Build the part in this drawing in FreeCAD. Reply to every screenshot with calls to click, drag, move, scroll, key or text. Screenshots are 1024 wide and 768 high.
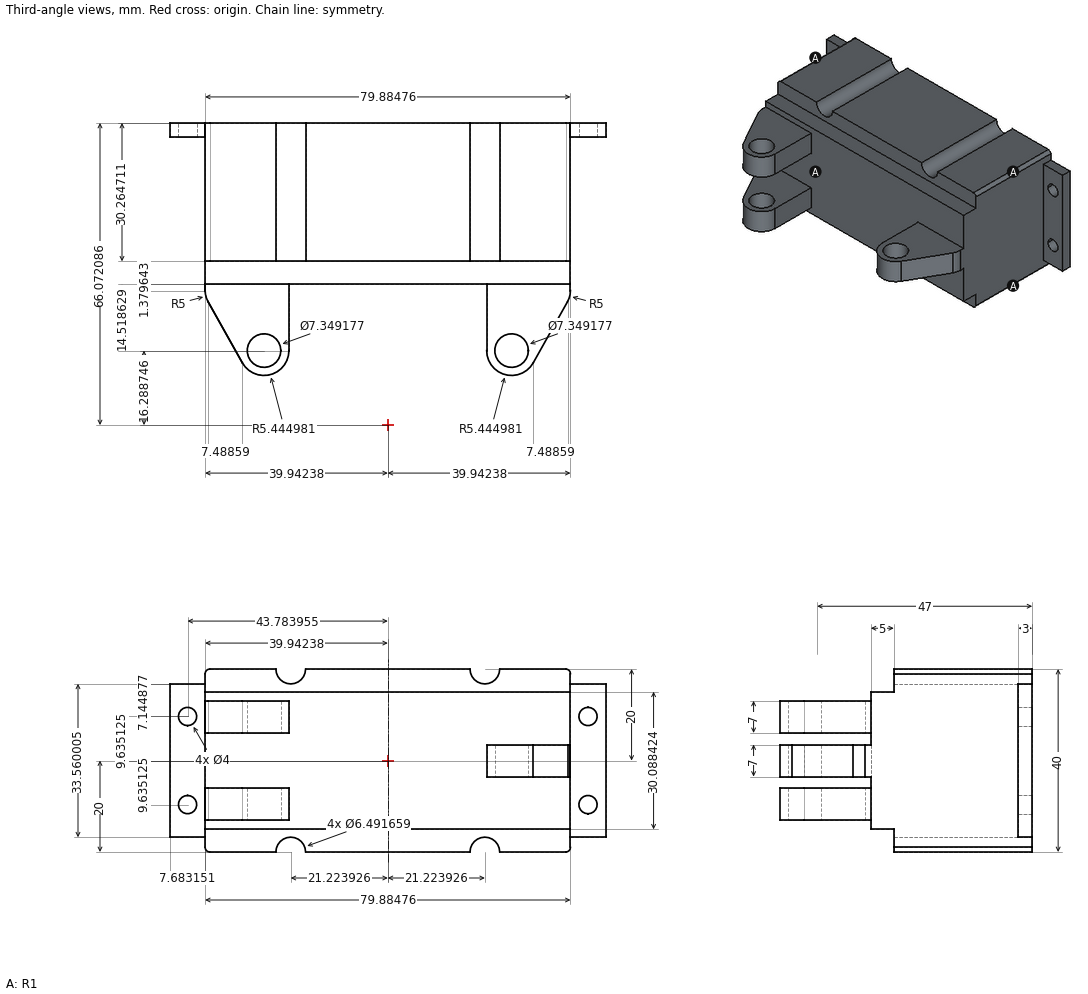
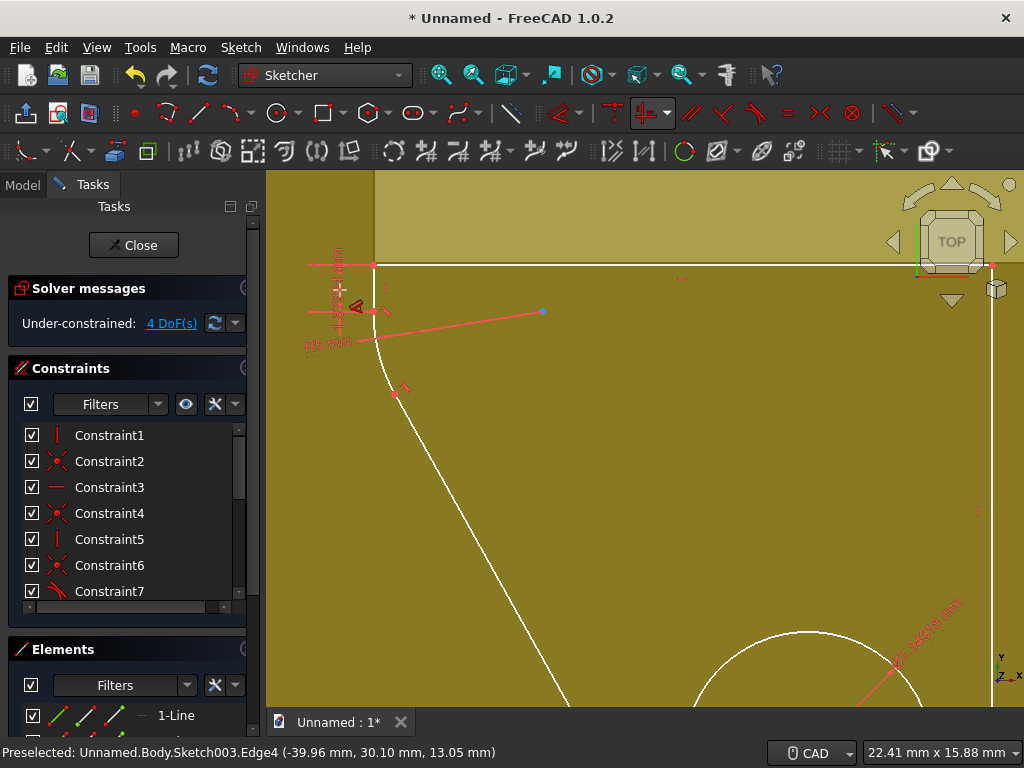
click(471, 530)
click(521, 360)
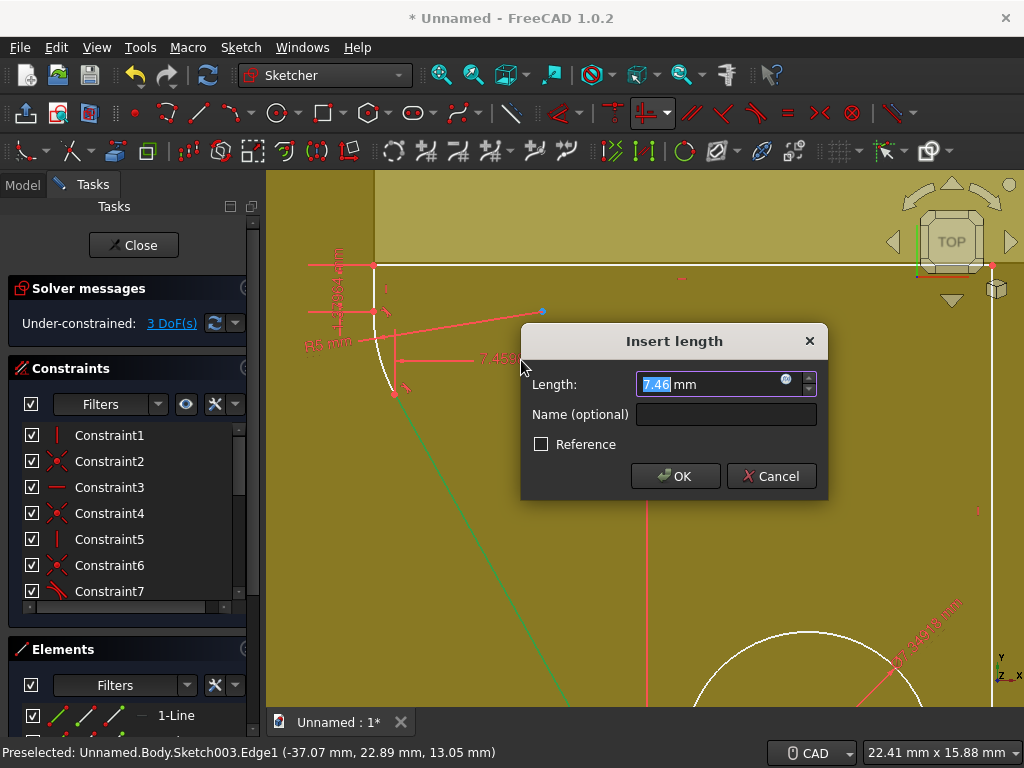
text(7.48859)
key(Return)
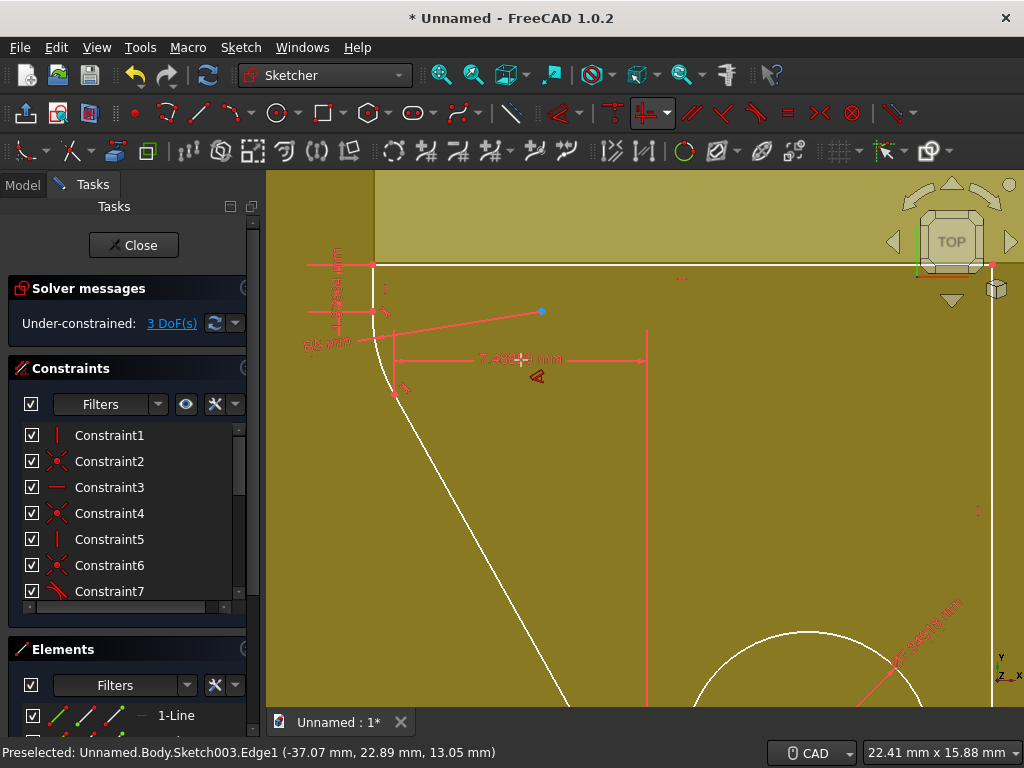
scroll(373, 290, down, 6)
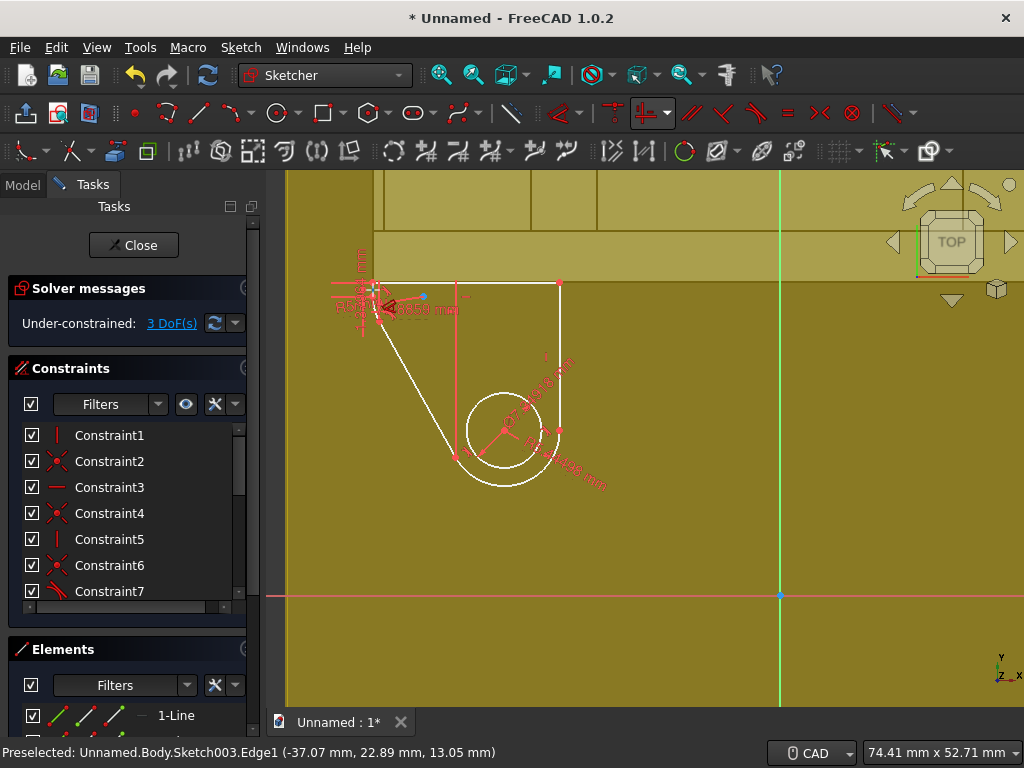
click(560, 386)
click(526, 357)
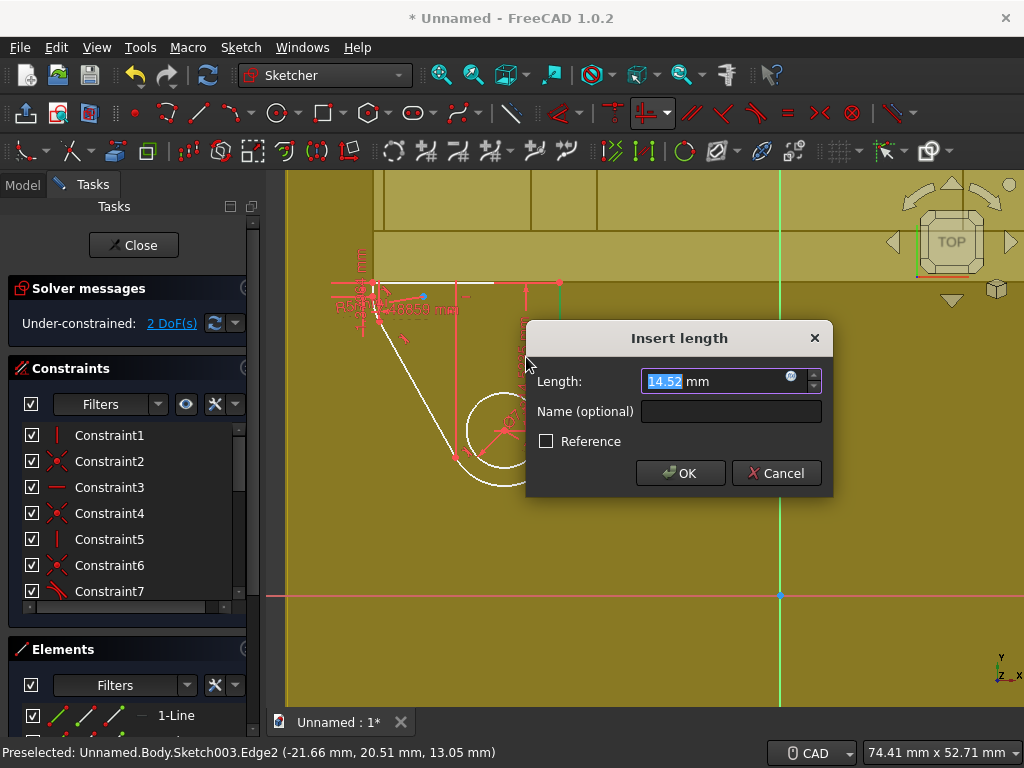
text(14.518629)
key(Return)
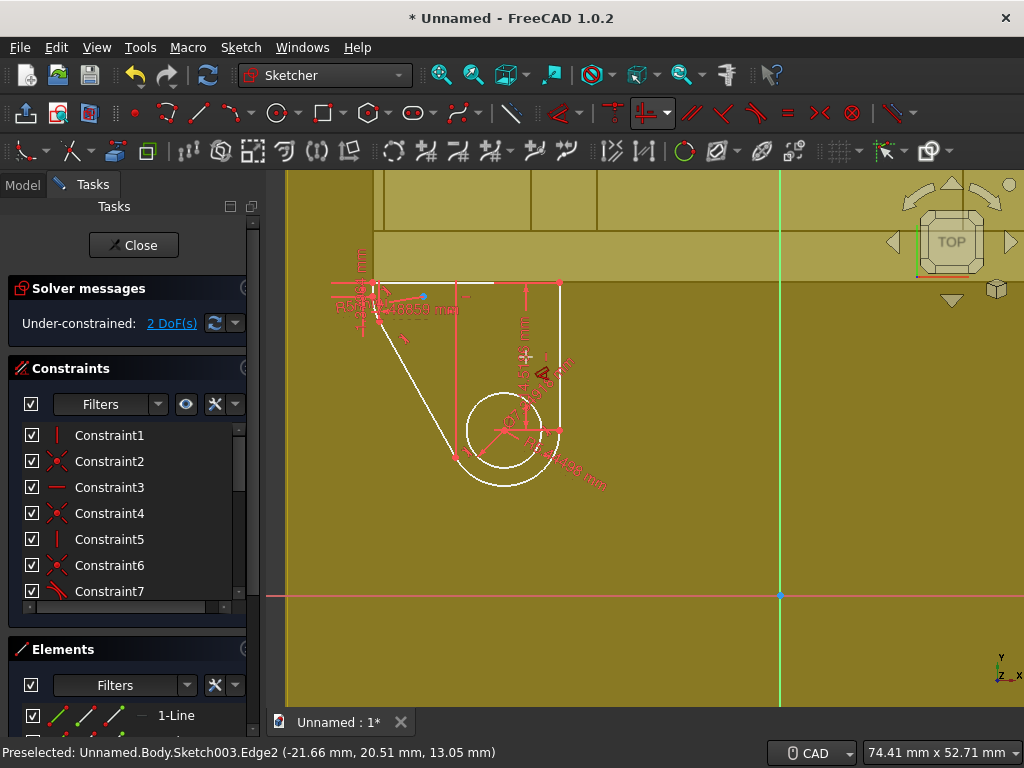
click(373, 283)
click(577, 630)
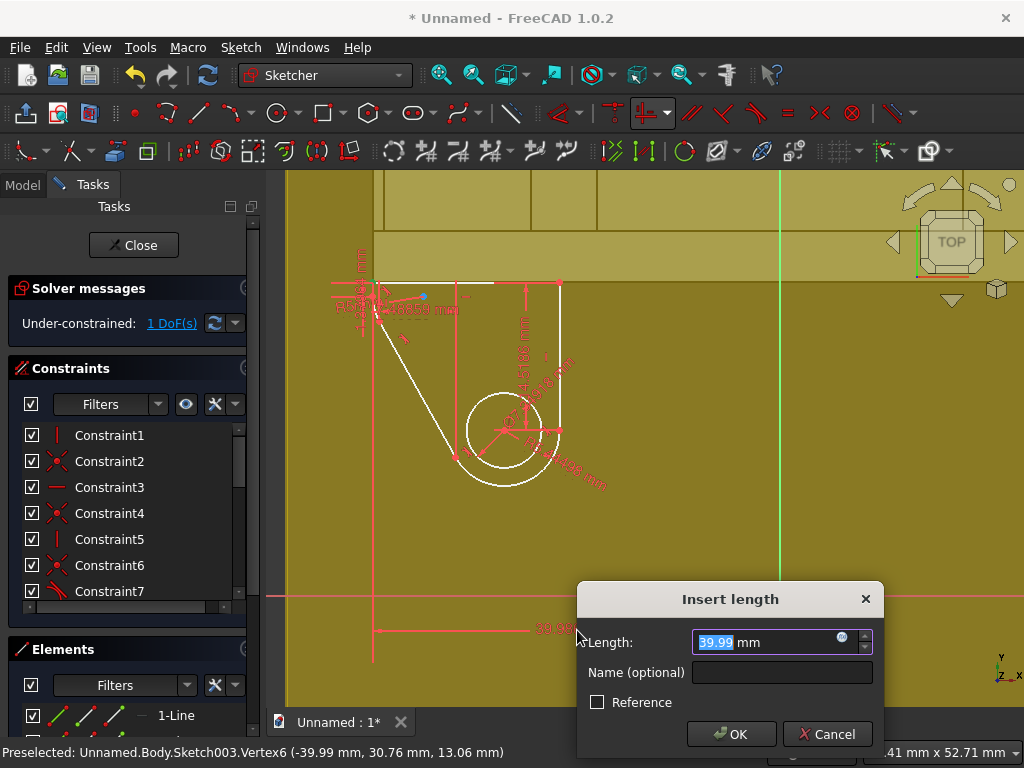
text(39.94238)
key(Return)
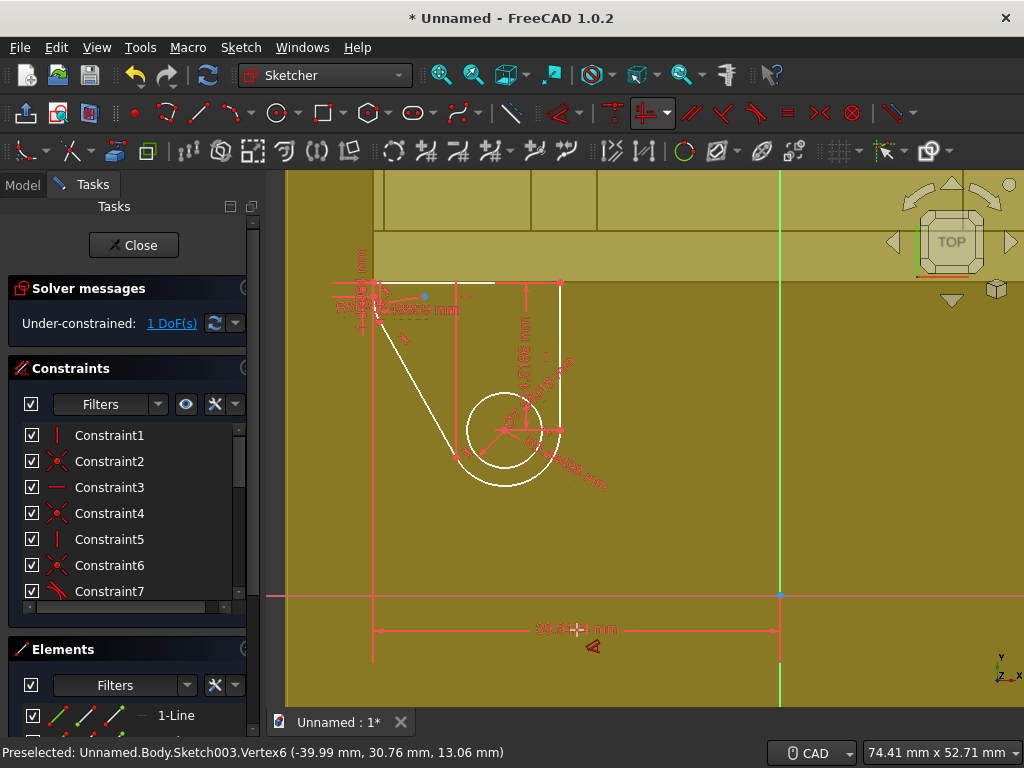
click(505, 430)
click(814, 513)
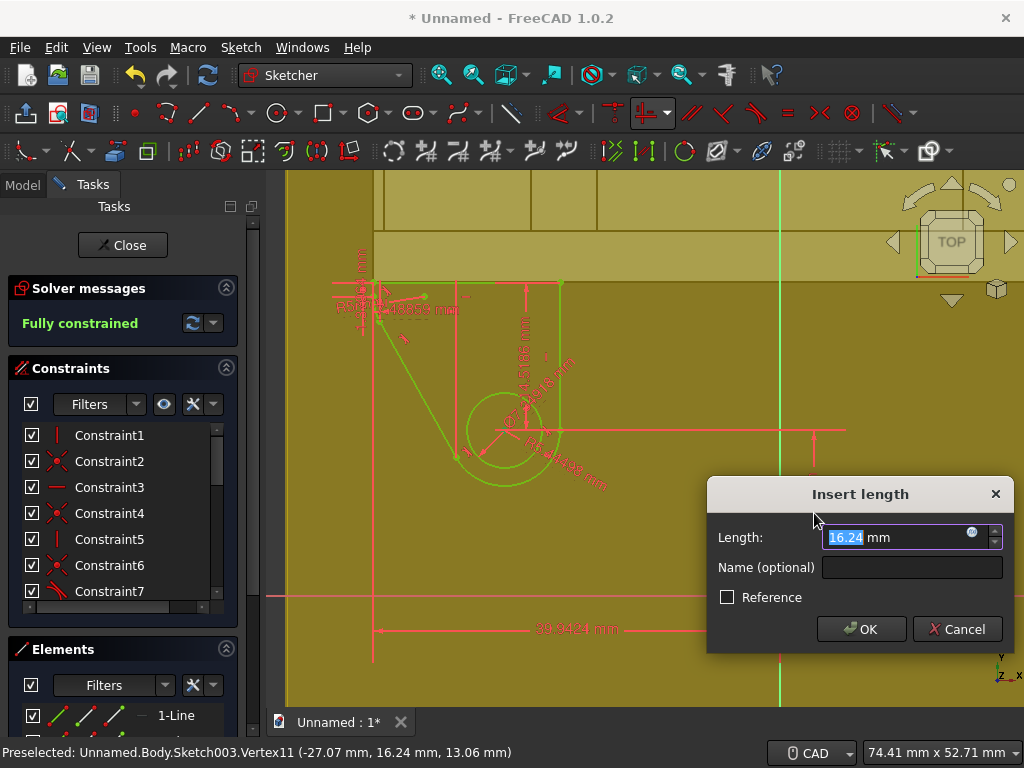
text(16.288746)
key(Return)
key(Escape)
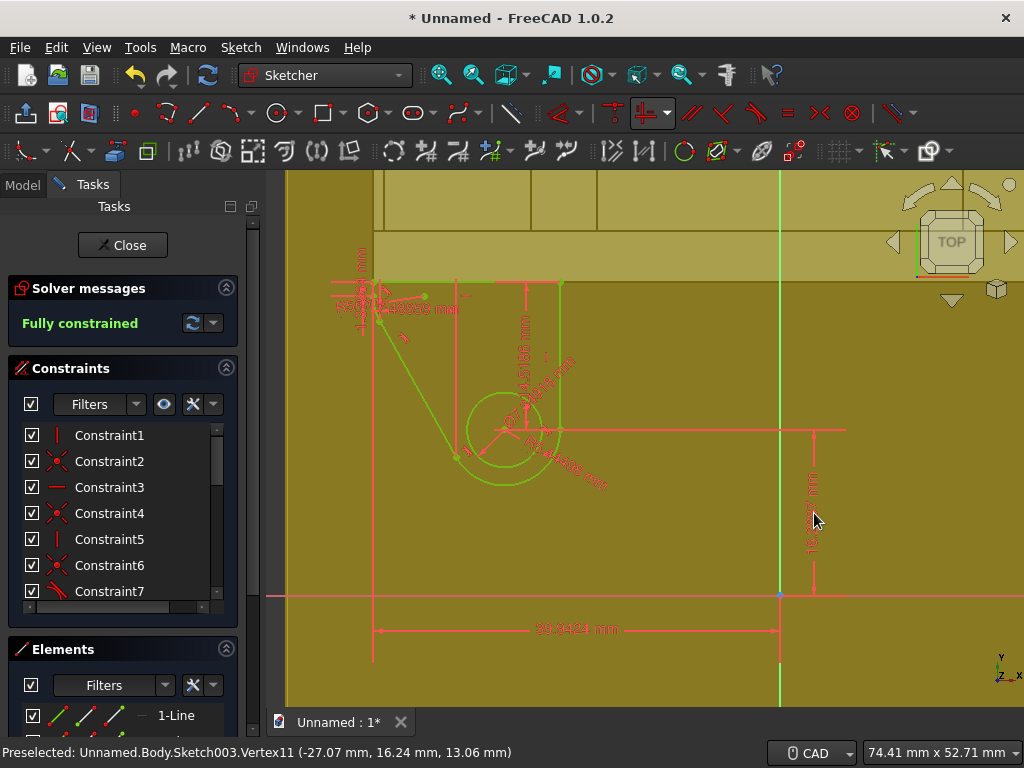
click(123, 245)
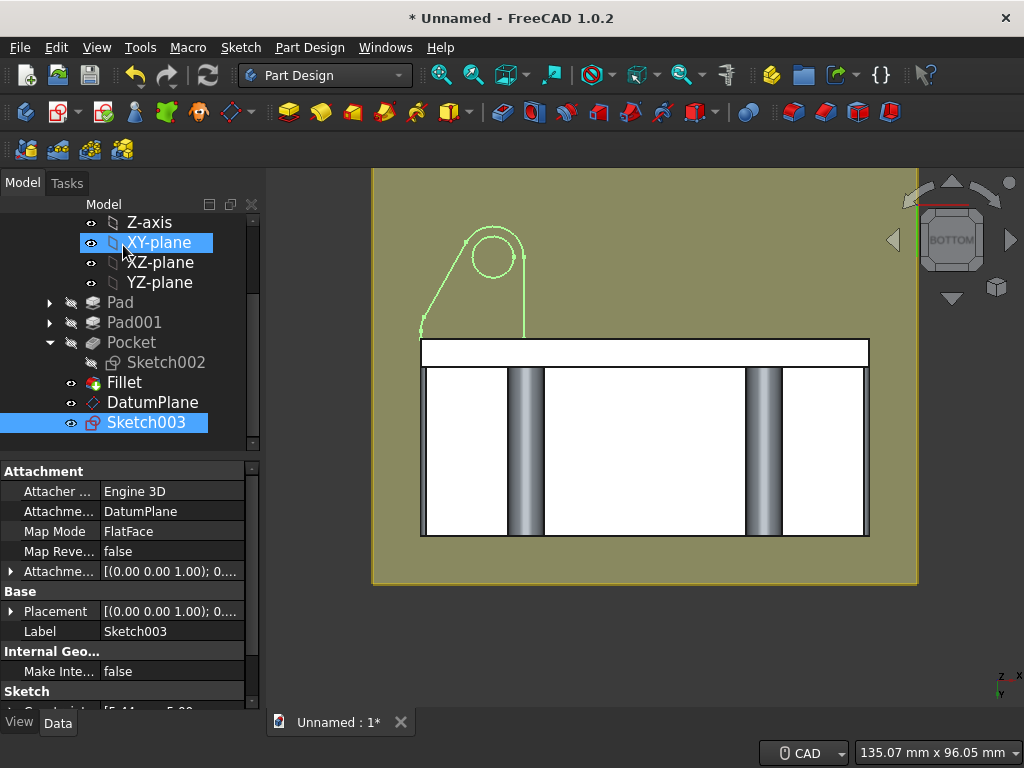
click(290, 112)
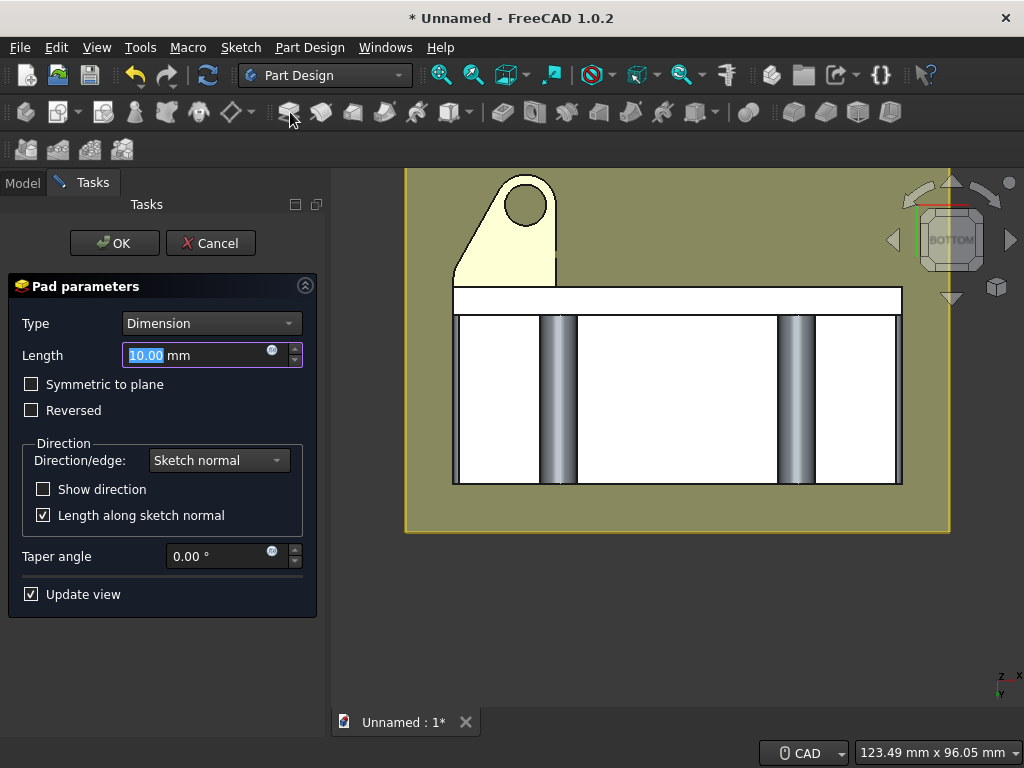
text(7)
key(Tab)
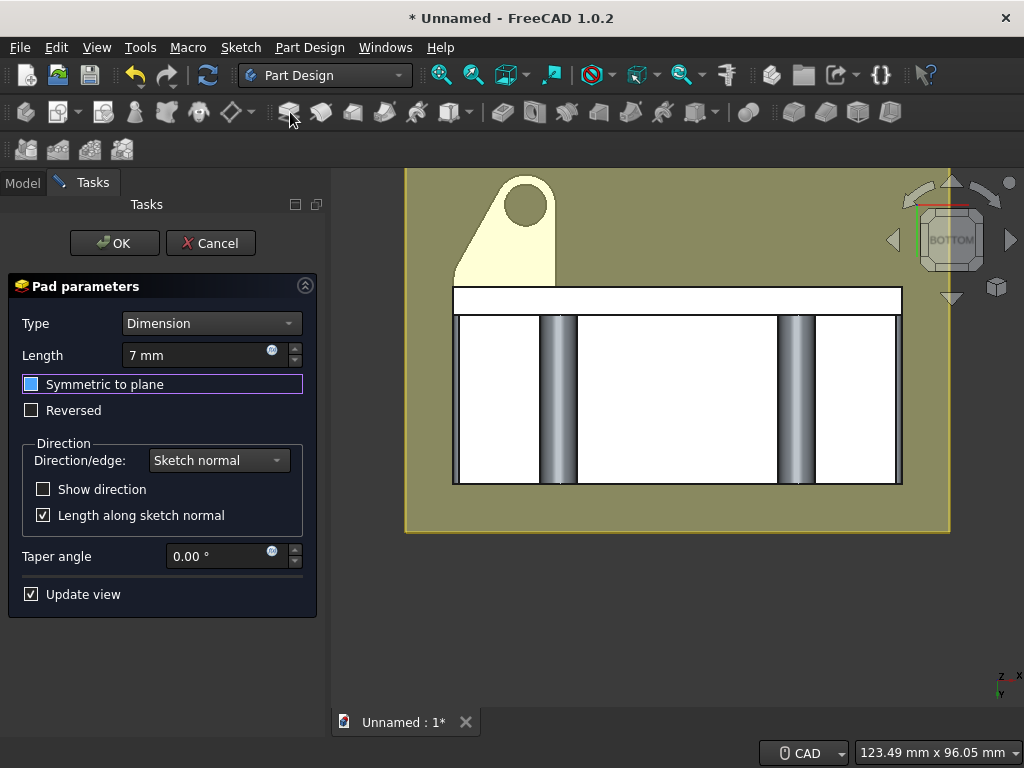
click(30, 410)